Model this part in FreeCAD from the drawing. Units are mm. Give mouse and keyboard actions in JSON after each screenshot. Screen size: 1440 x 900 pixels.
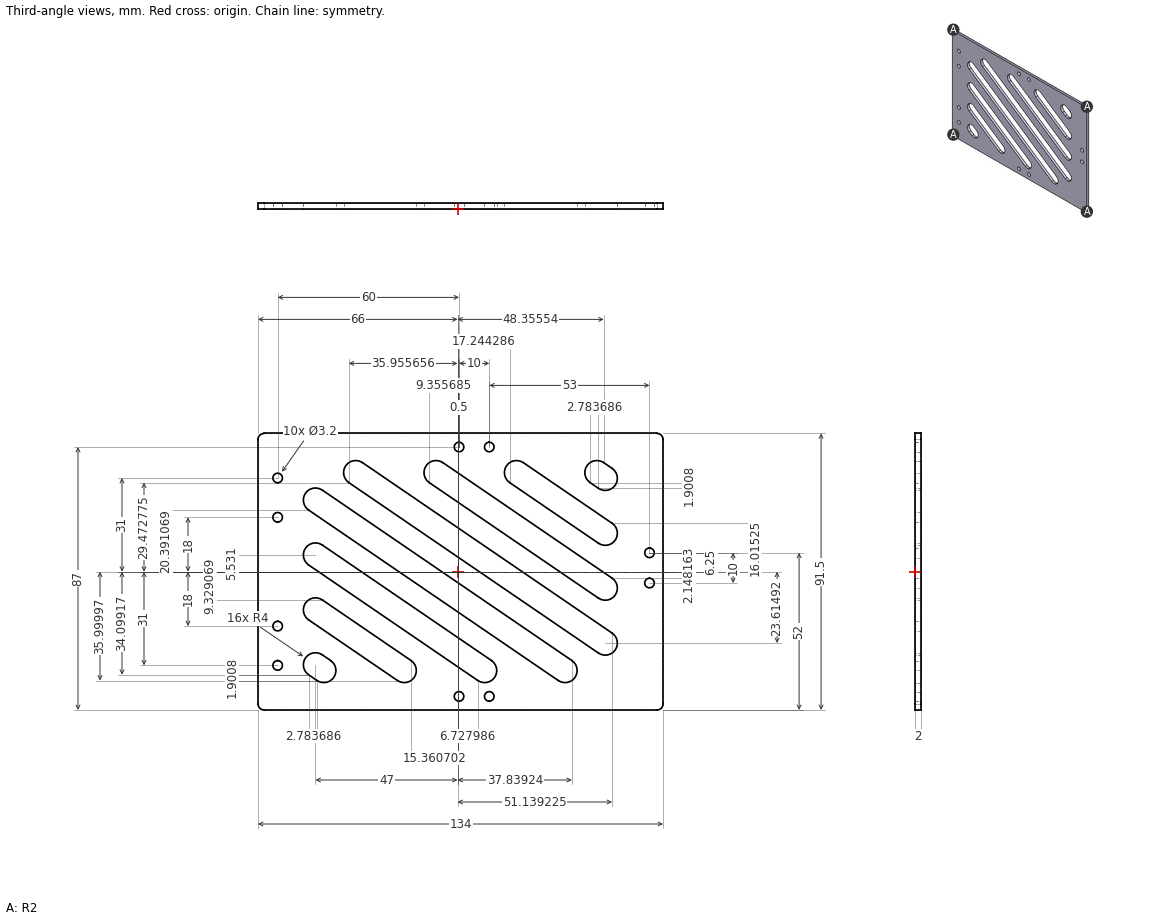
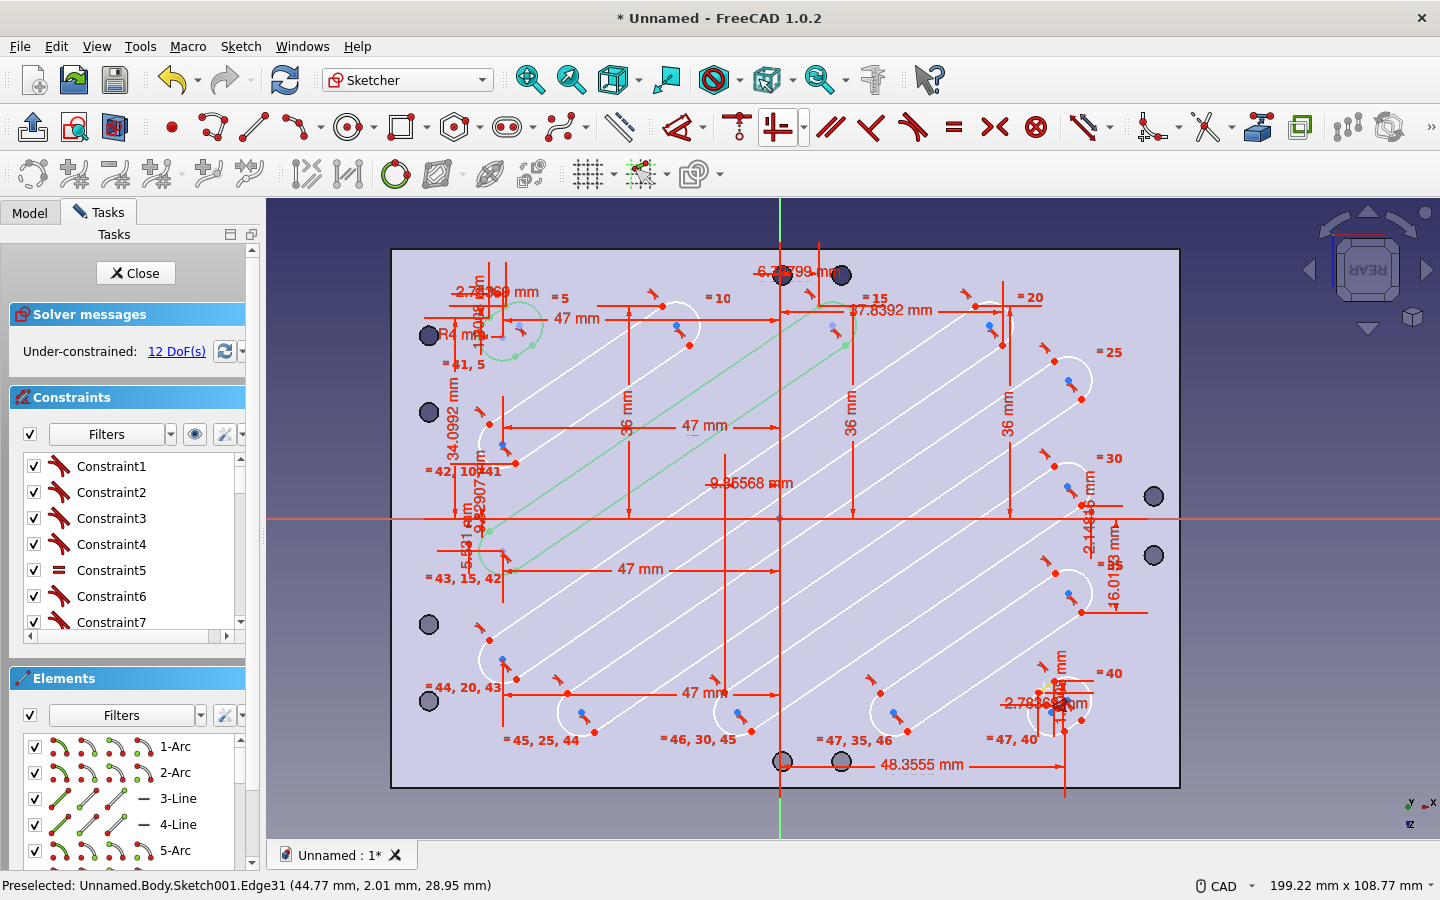
{"action": "left_click", "coordinate": [1068, 381]}
{"action": "left_click", "coordinate": [1102, 450]}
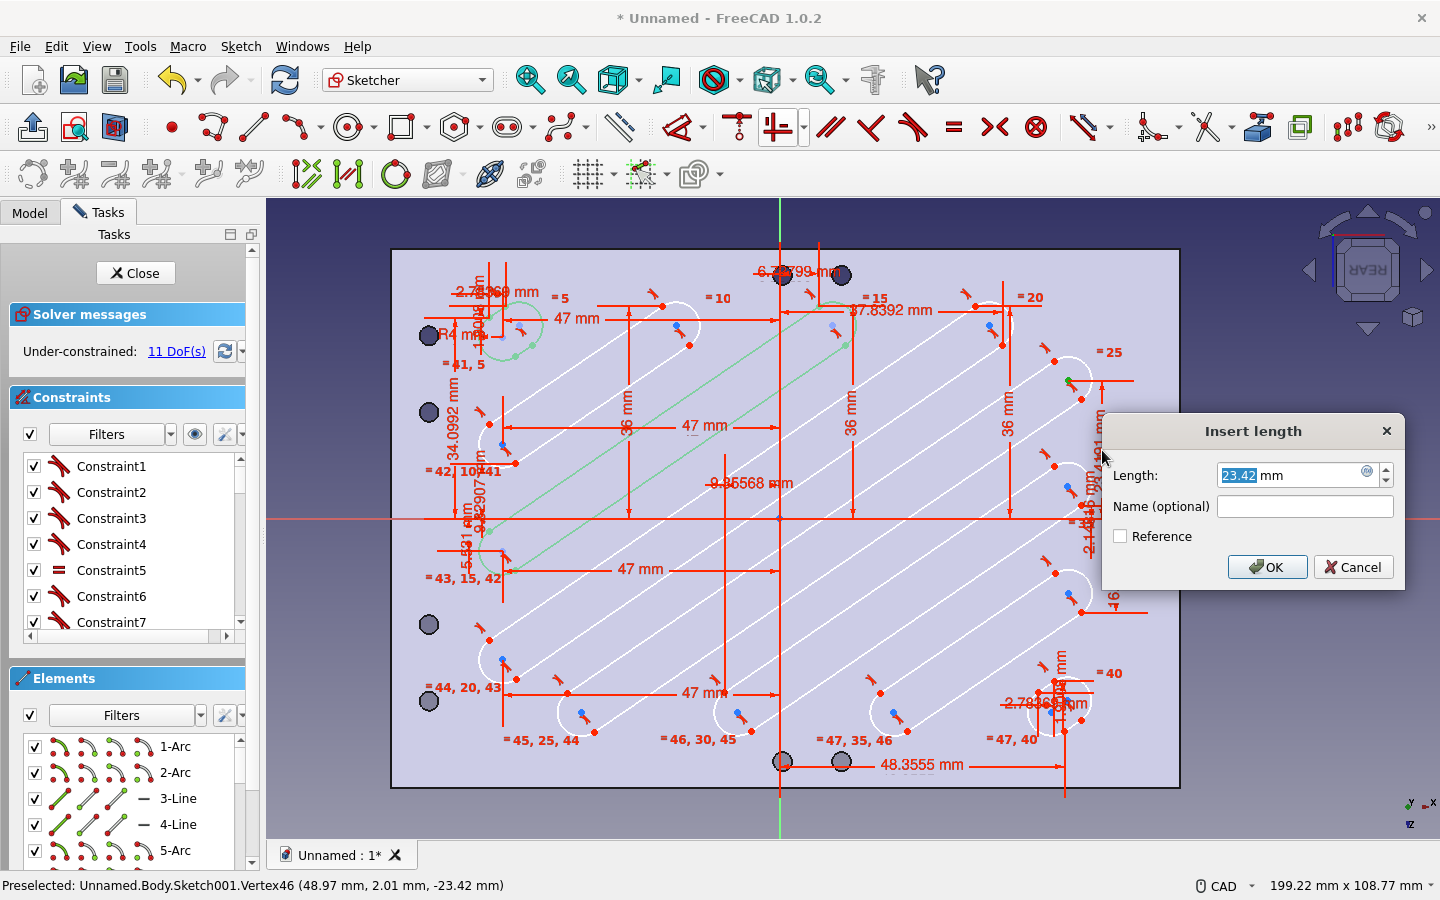
{"action": "type", "text": "23.61492"}
{"action": "key", "text": "Return"}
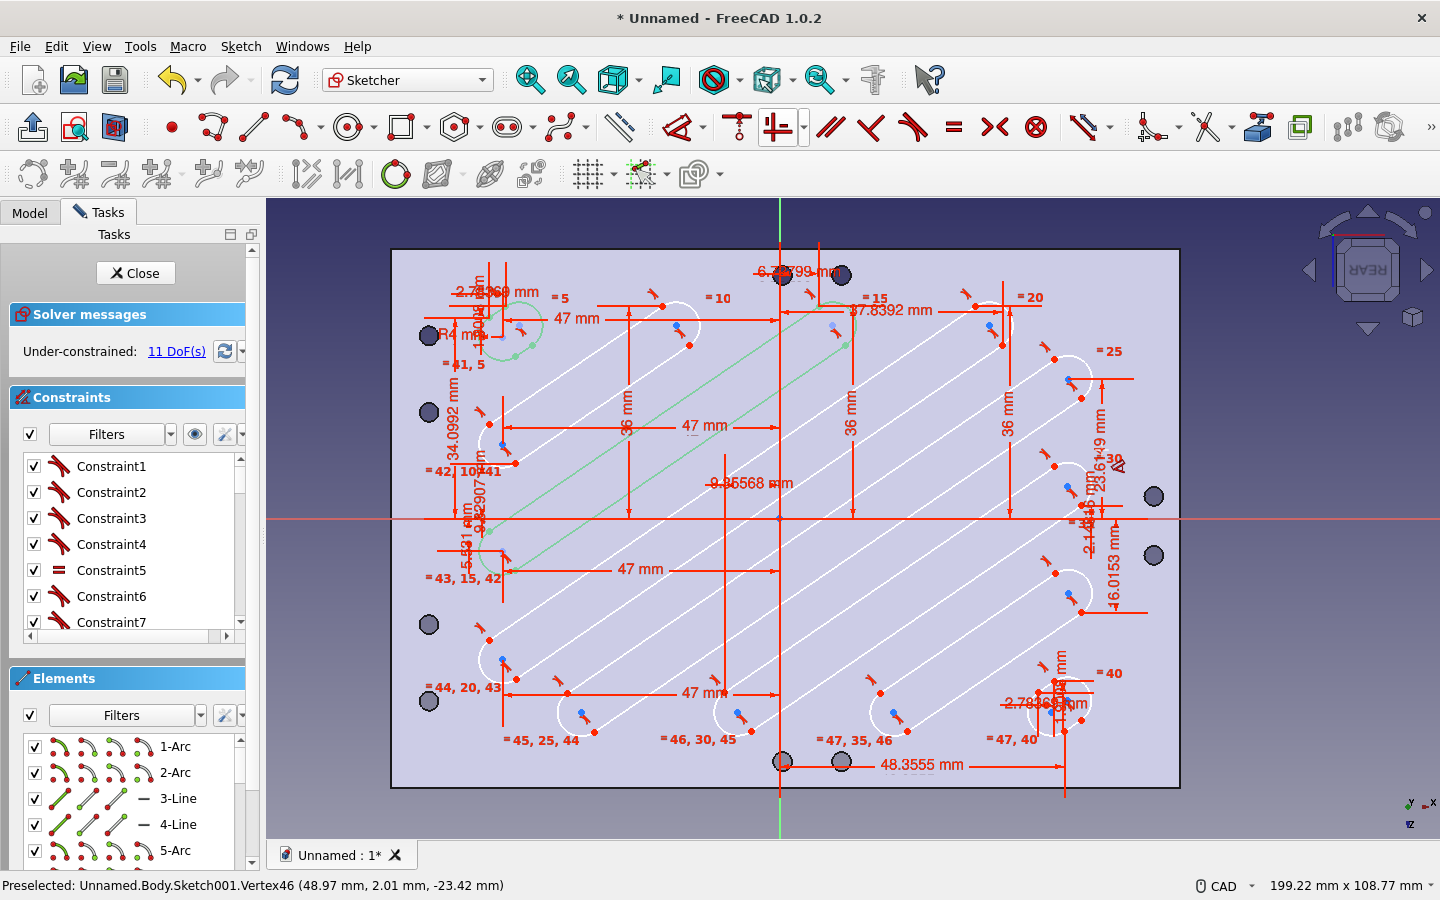
{"action": "left_click", "coordinate": [690, 345]}
{"action": "left_click", "coordinate": [735, 311]}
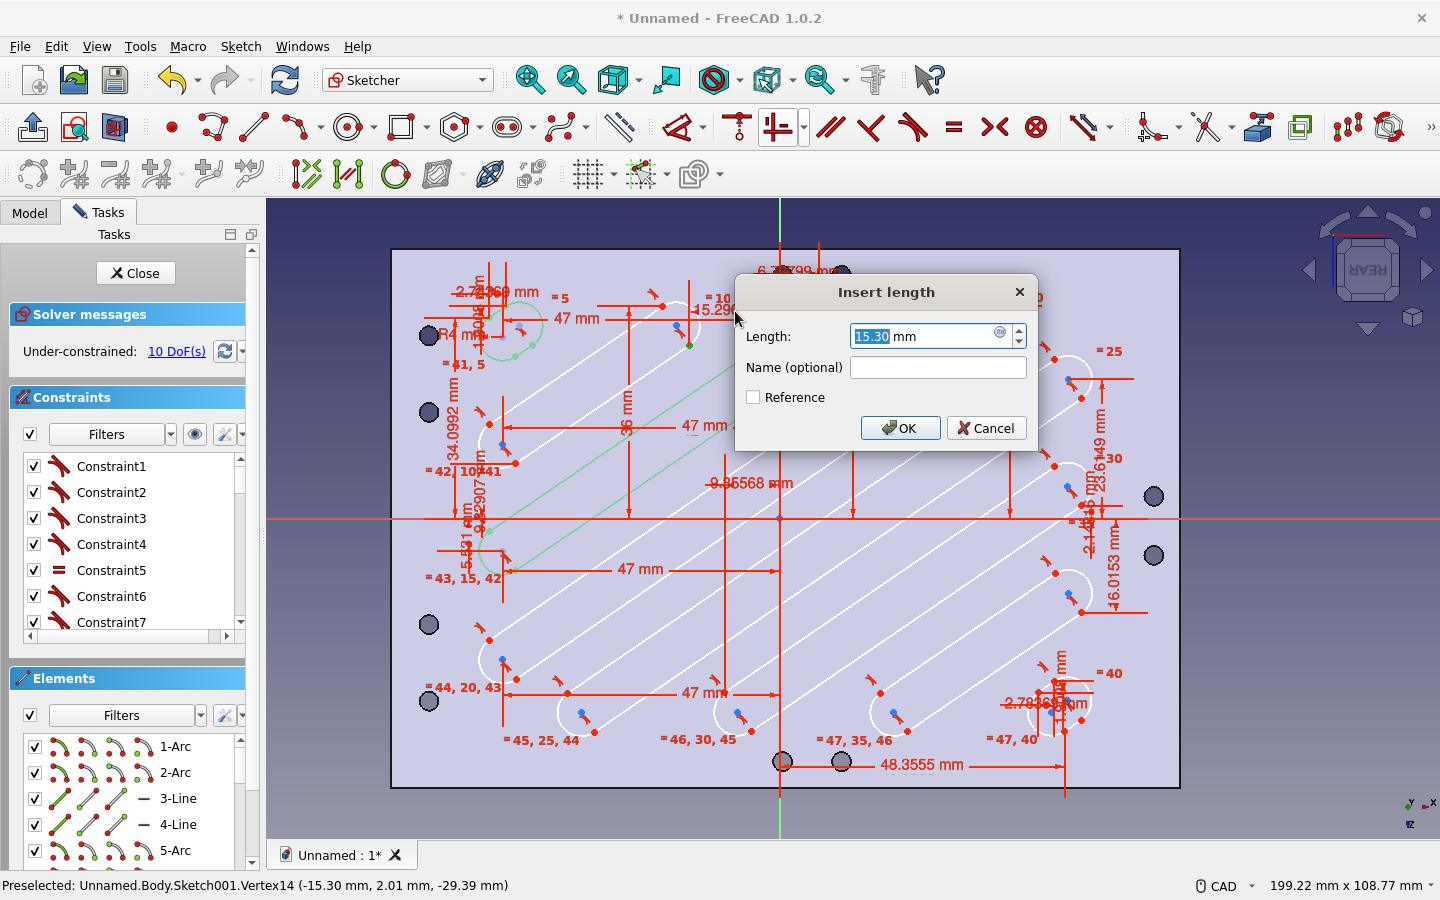
{"action": "type", "text": "15.360702"}
{"action": "key", "text": "Return"}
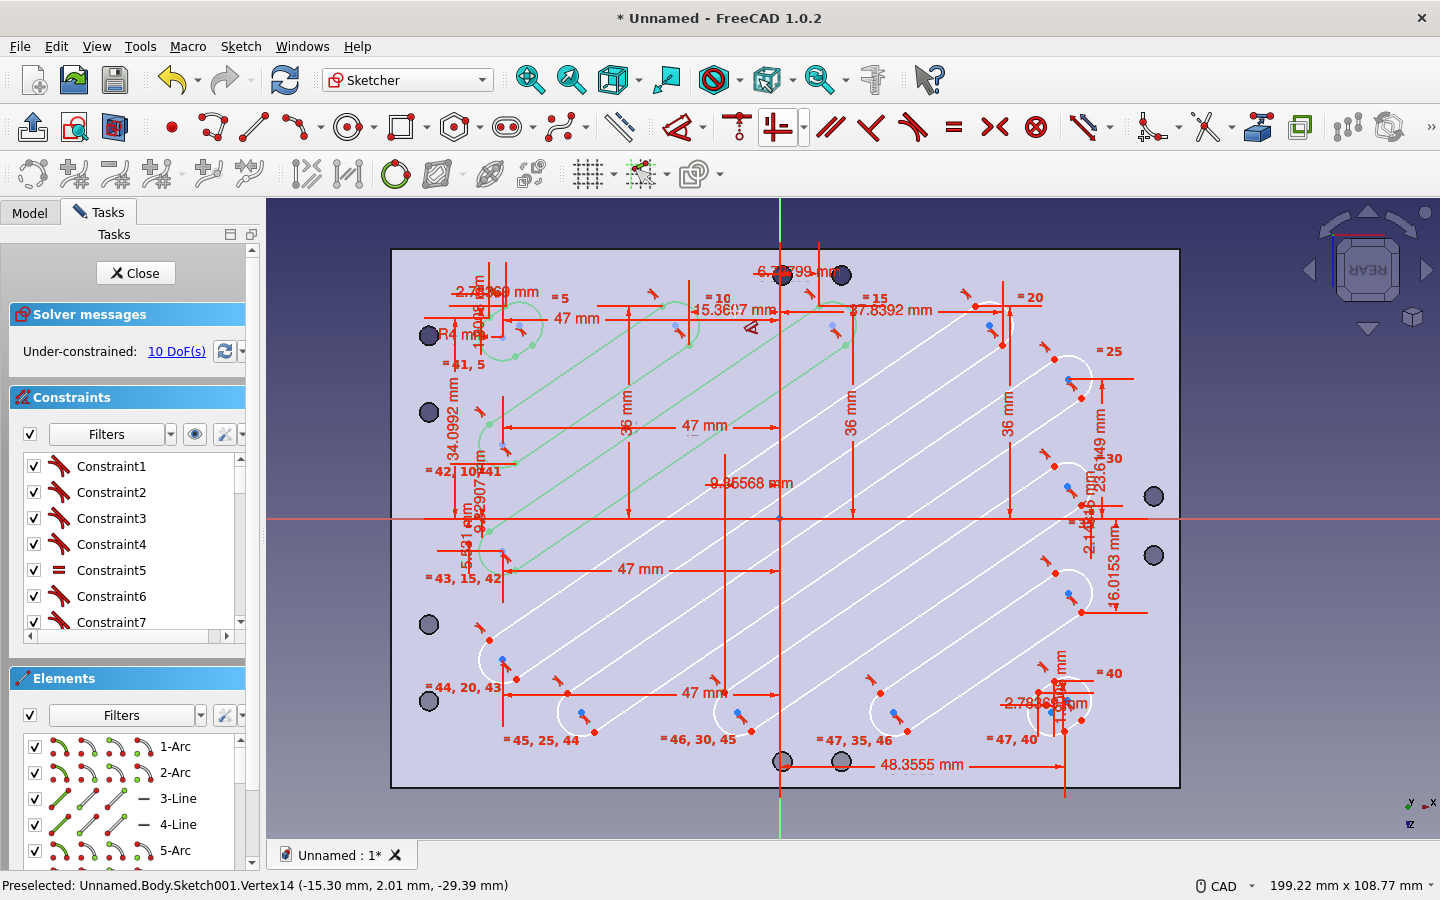
{"action": "left_click", "coordinate": [489, 640]}
{"action": "left_click", "coordinate": [455, 579]}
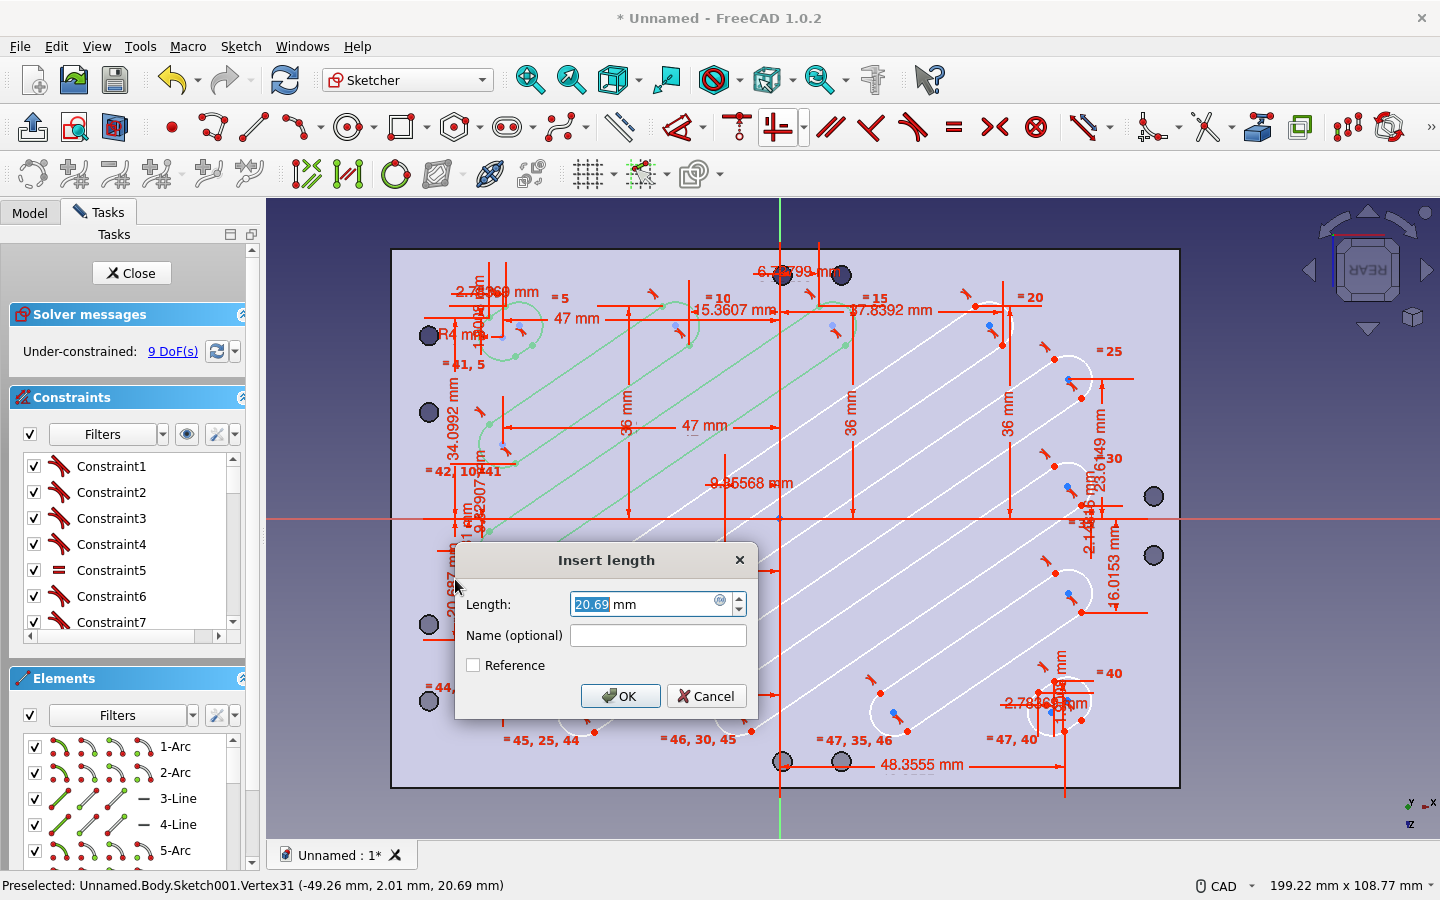
{"action": "type", "text": "20.391069"}
{"action": "key", "text": "Return"}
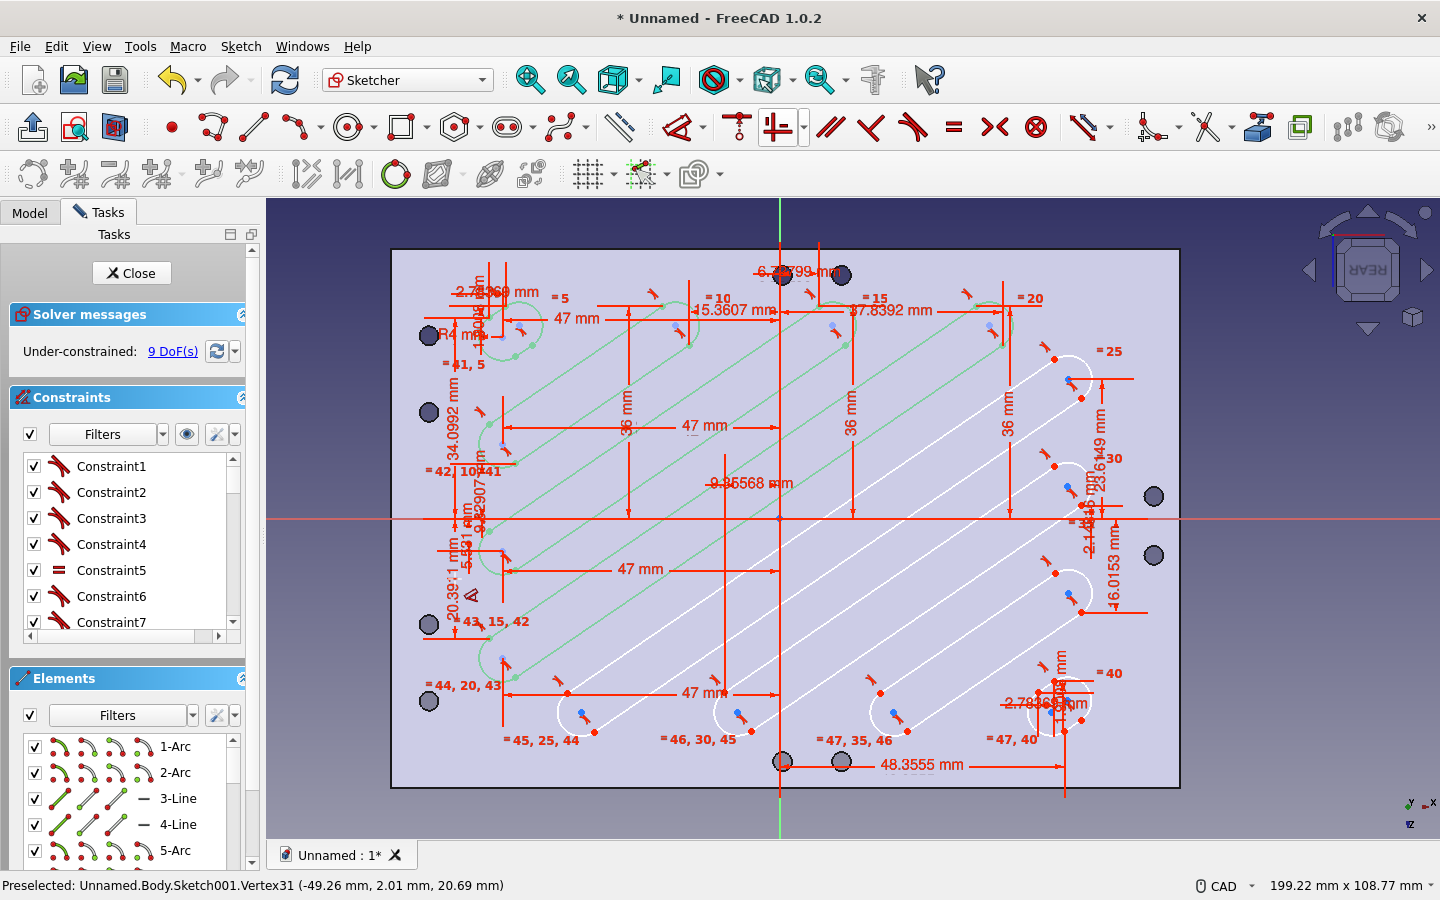
{"action": "left_click", "coordinate": [568, 693]}
{"action": "left_click", "coordinate": [674, 727]}